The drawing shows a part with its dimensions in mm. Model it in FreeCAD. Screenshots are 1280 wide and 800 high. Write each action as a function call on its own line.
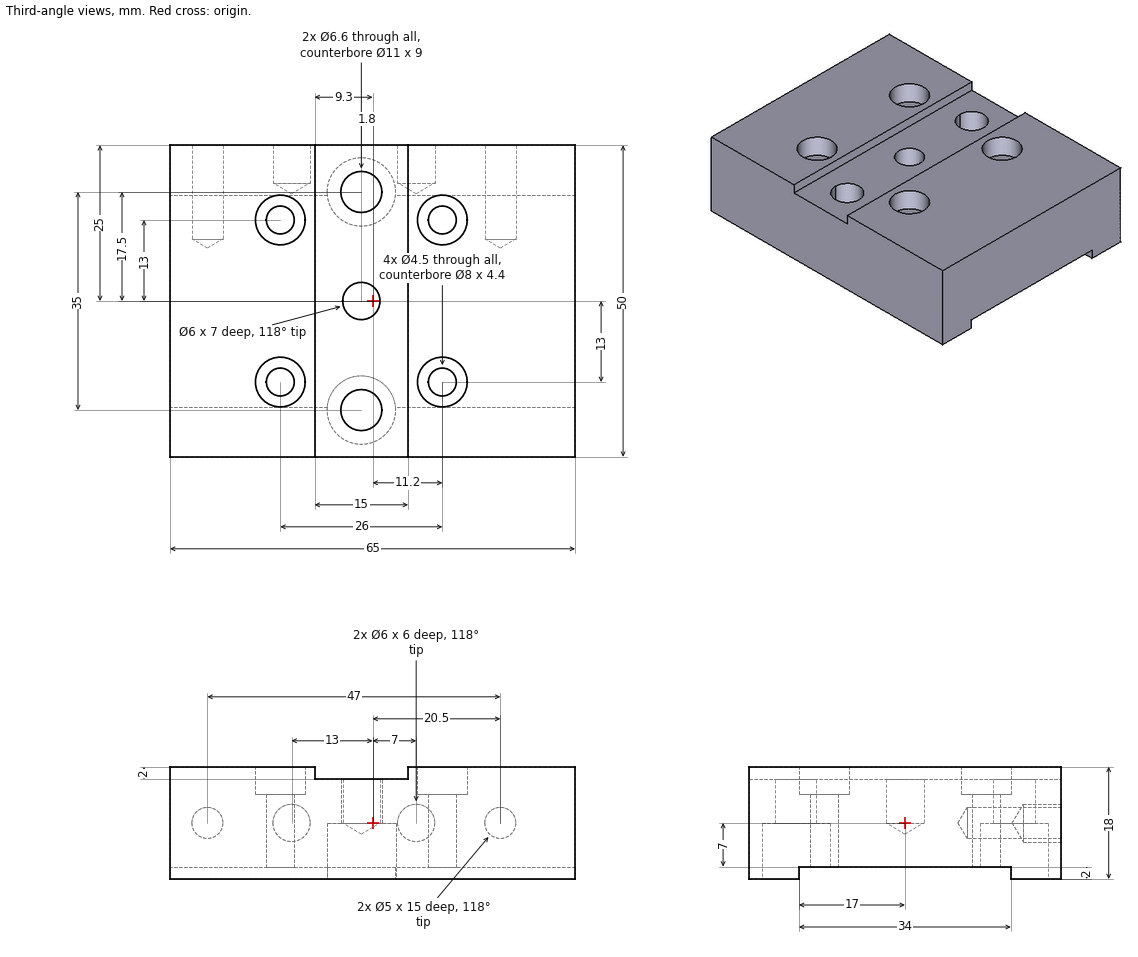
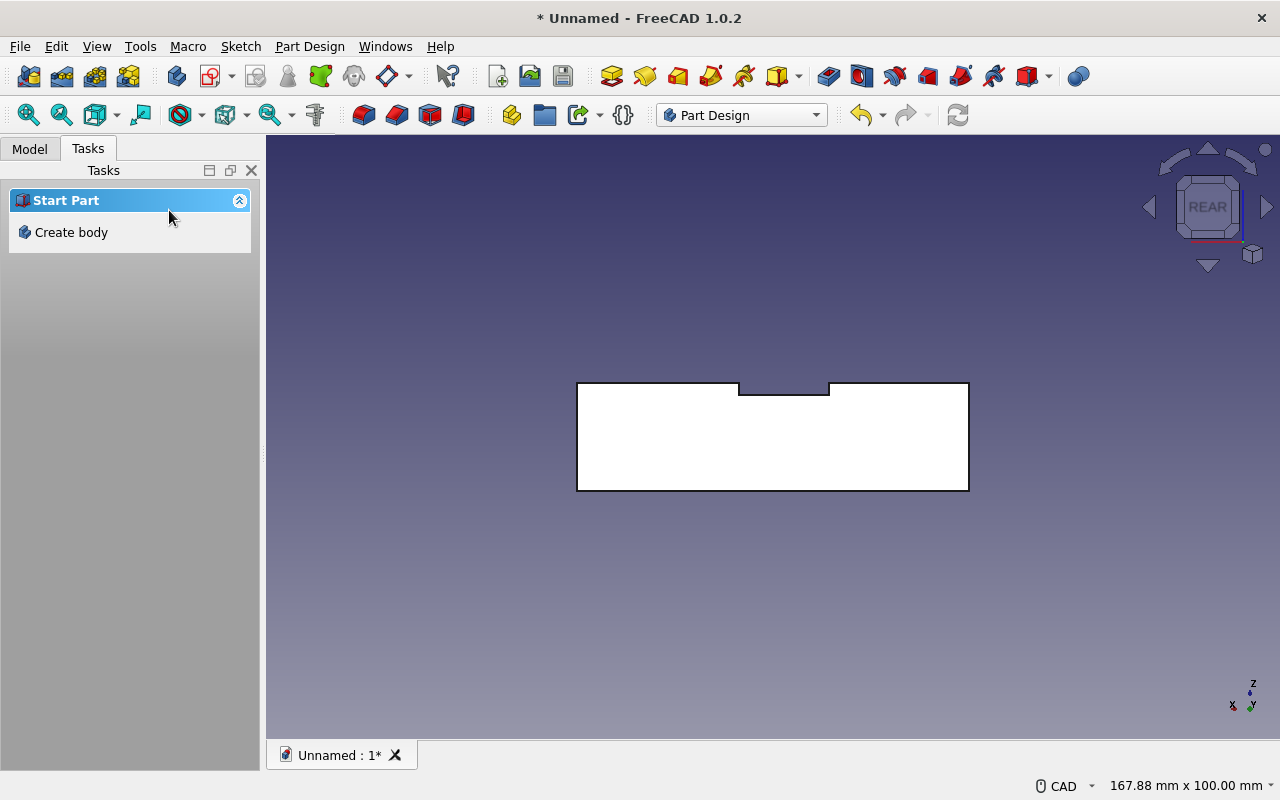
key(v)
key(f)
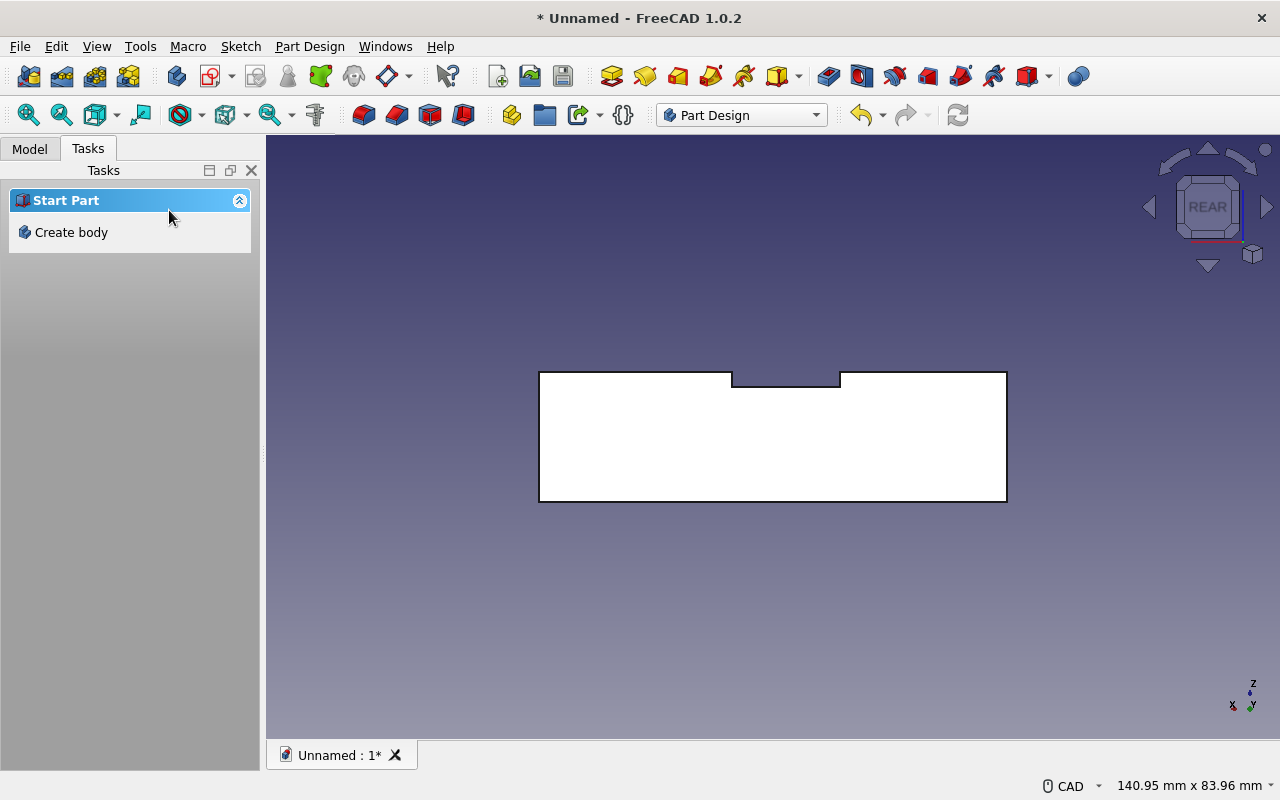
click(639, 436)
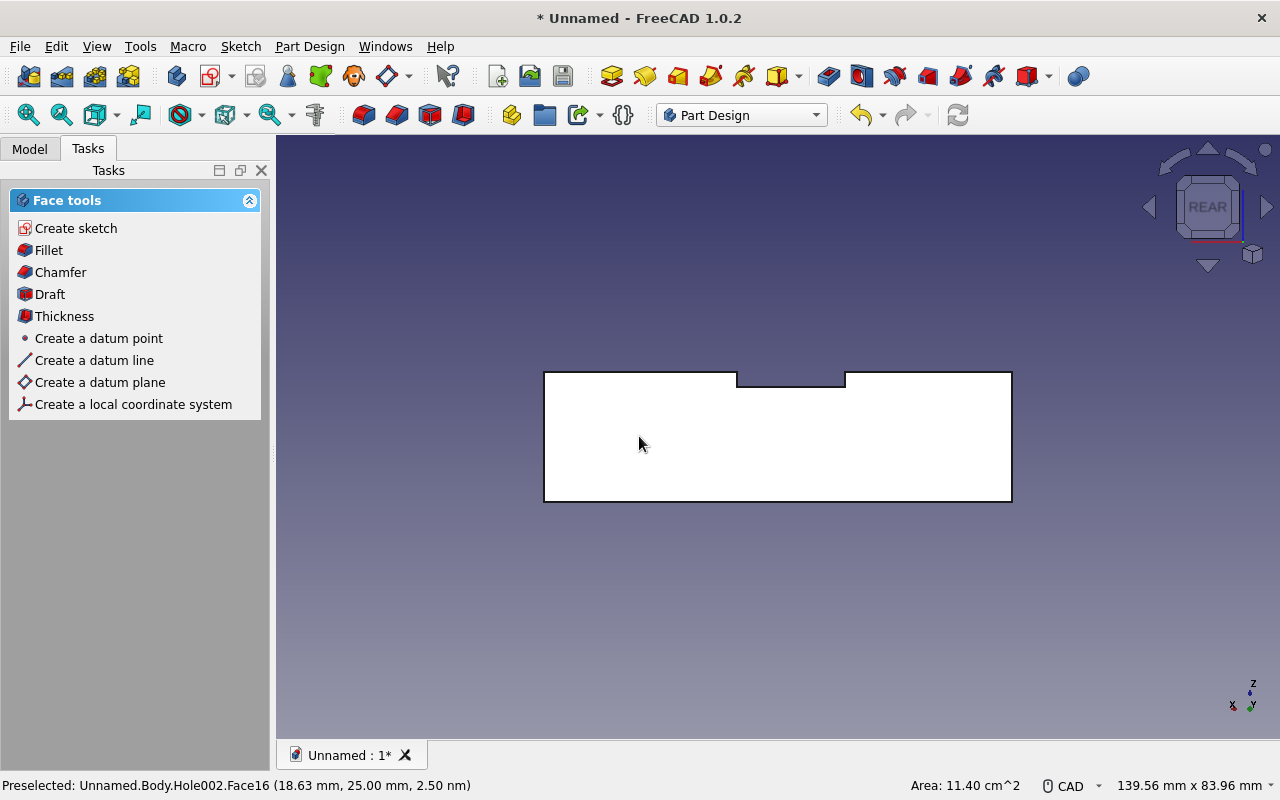
click(210, 76)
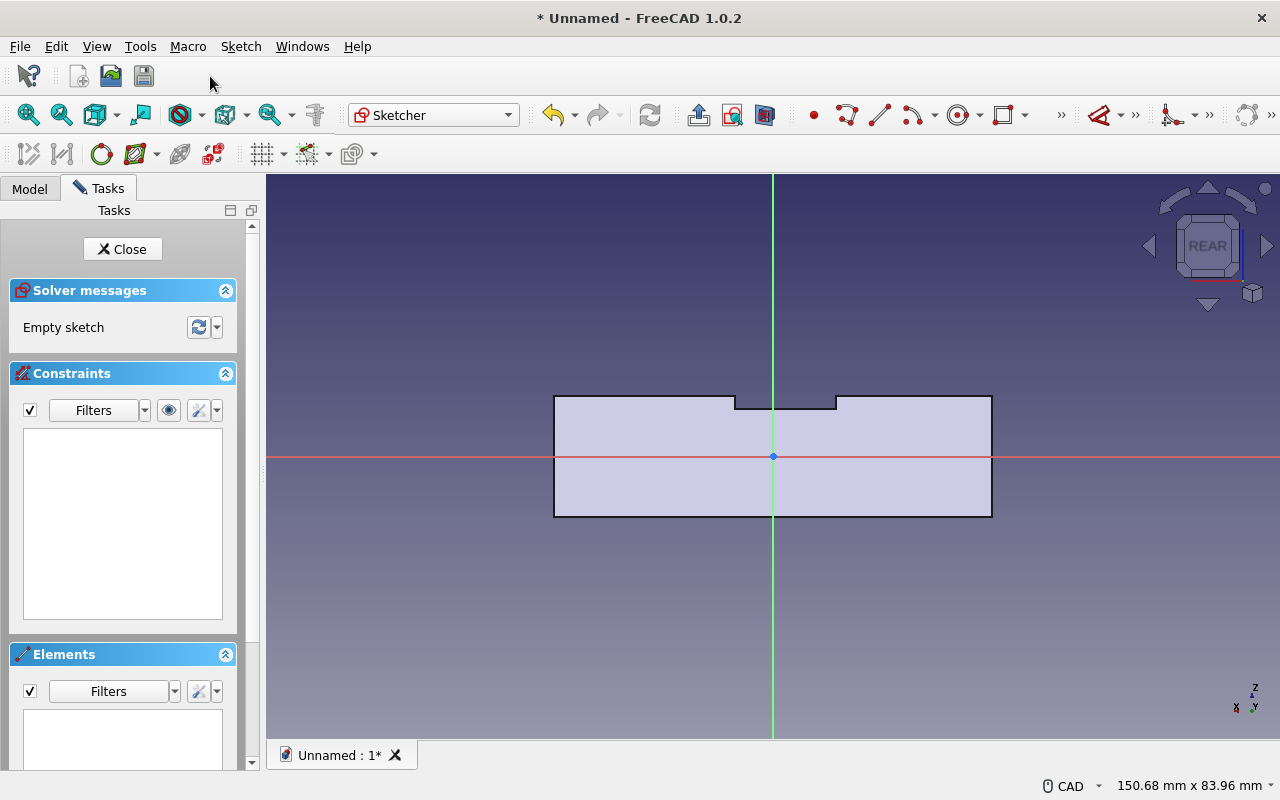
scroll(901, 456, up, 3)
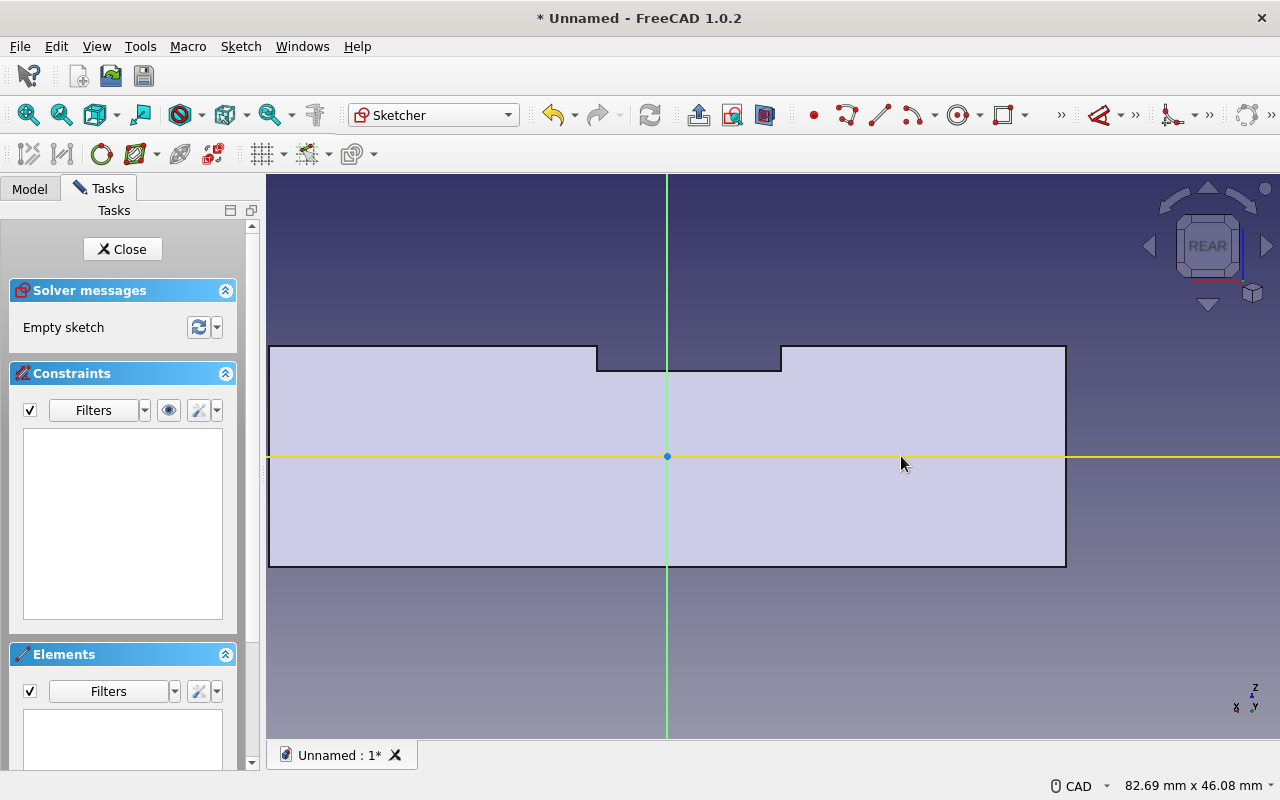
click(958, 116)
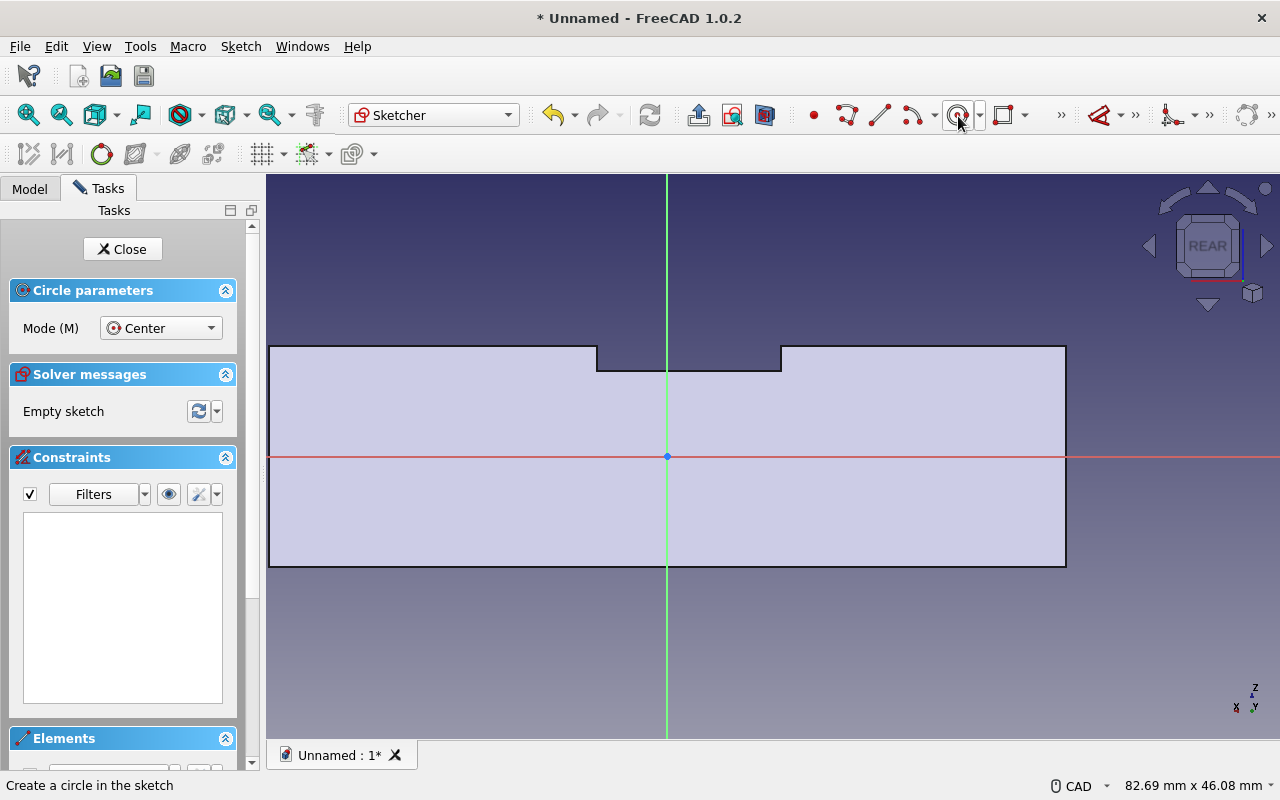
click(416, 456)
move(438, 435)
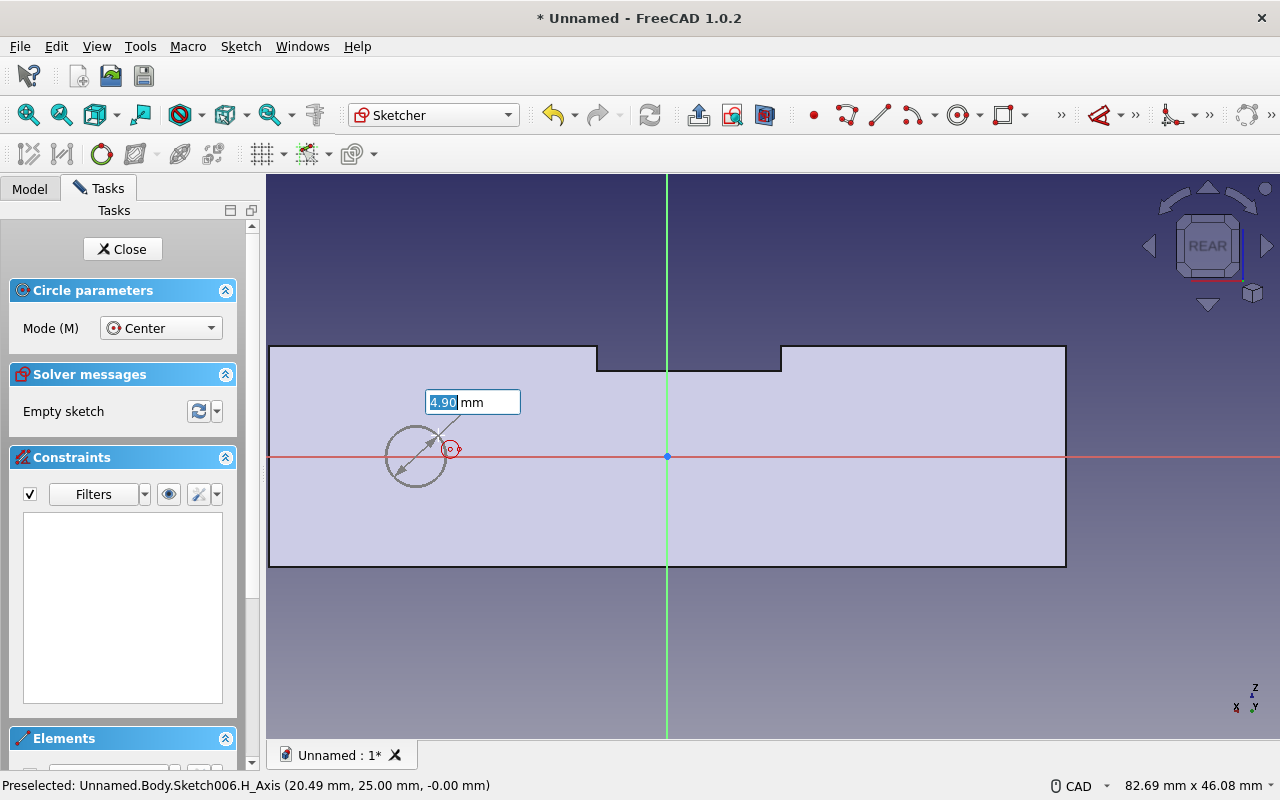
text(5)
key(Return)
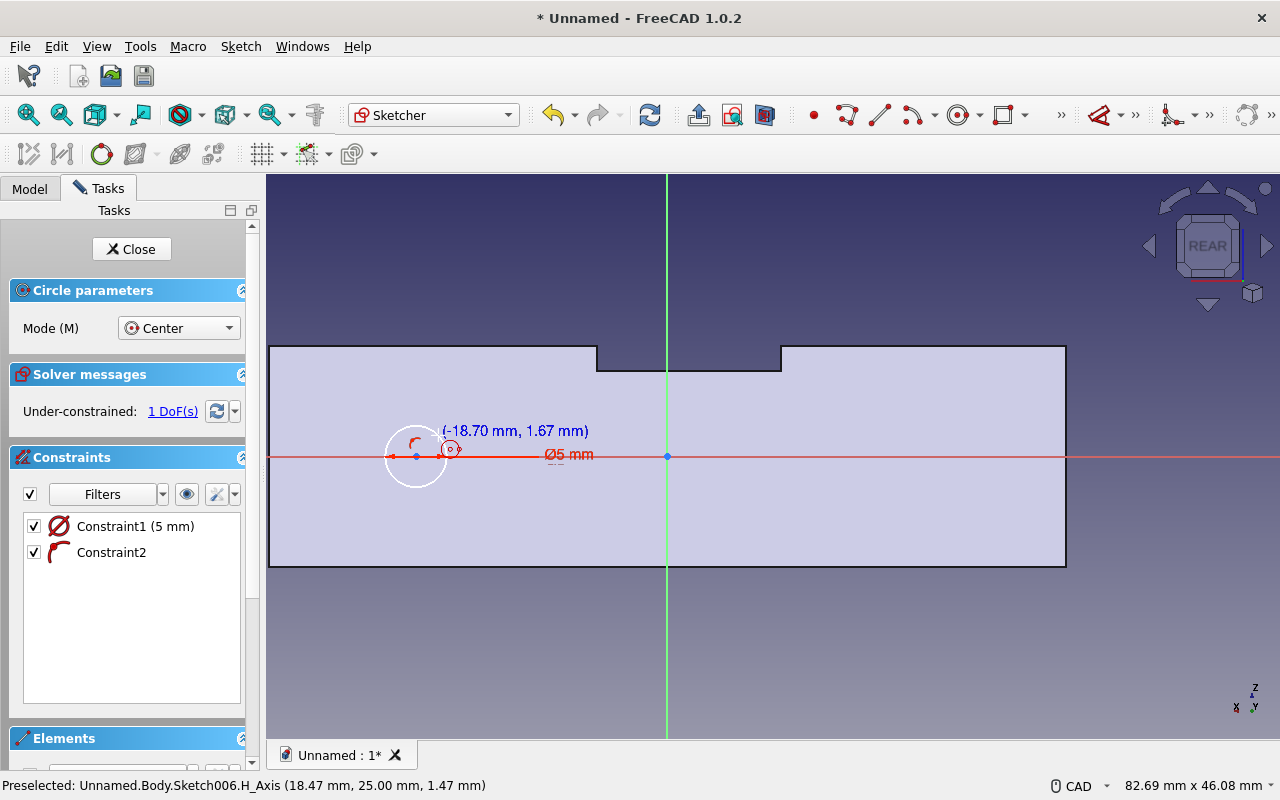
click(992, 456)
move(1014, 435)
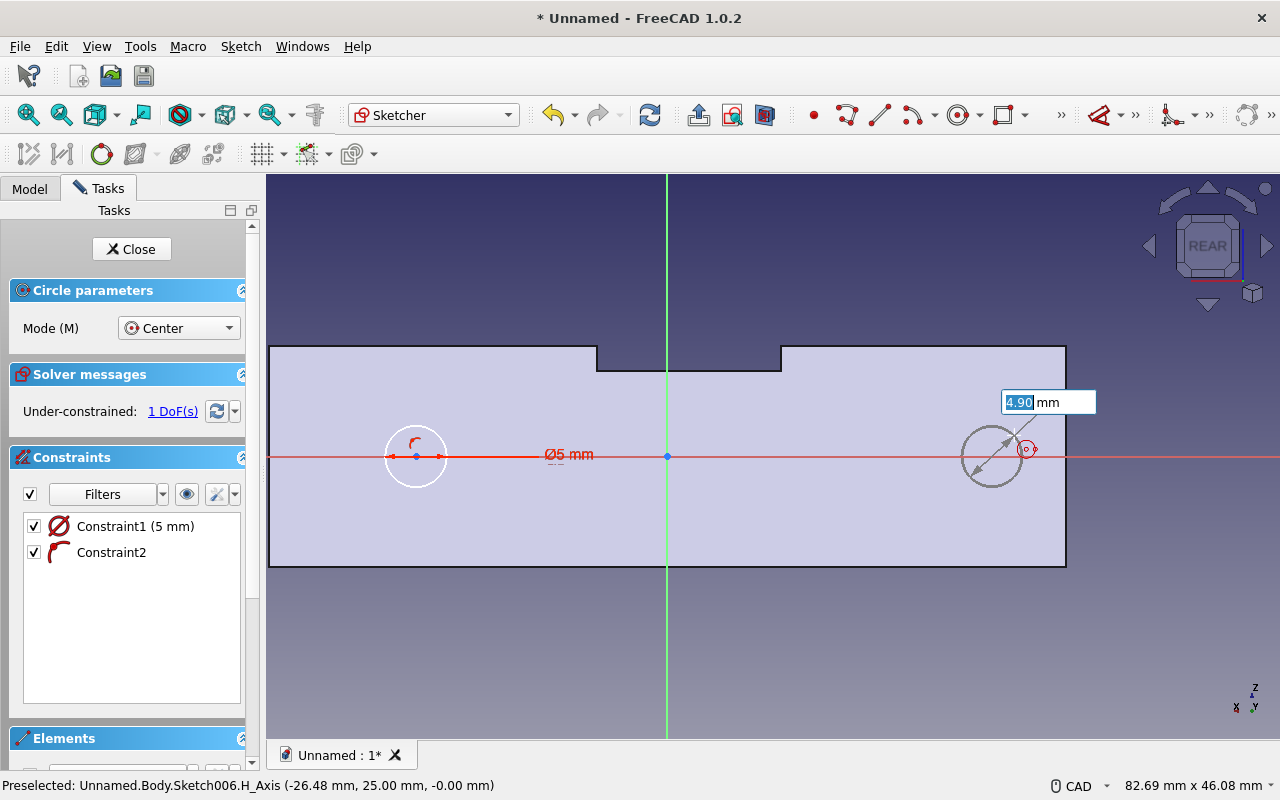
text(5)
key(Return)
key(Escape)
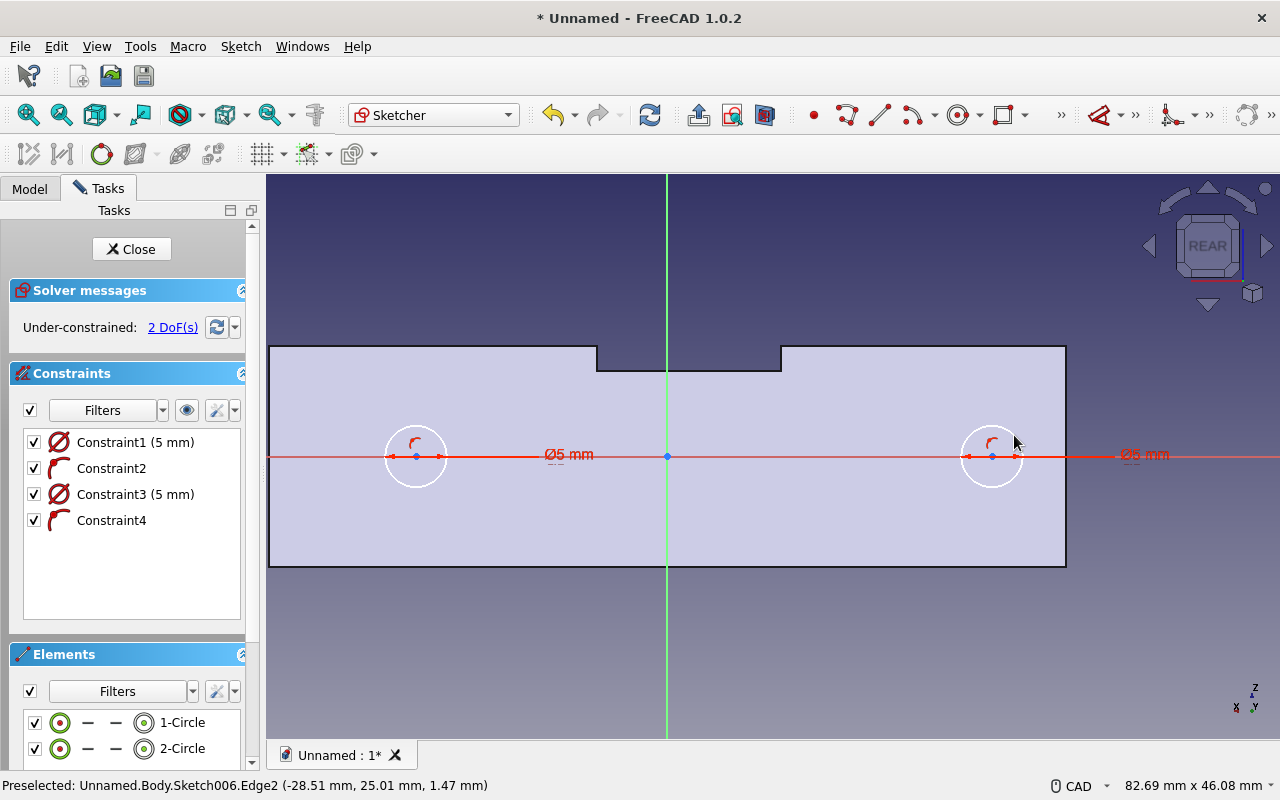
key(d)